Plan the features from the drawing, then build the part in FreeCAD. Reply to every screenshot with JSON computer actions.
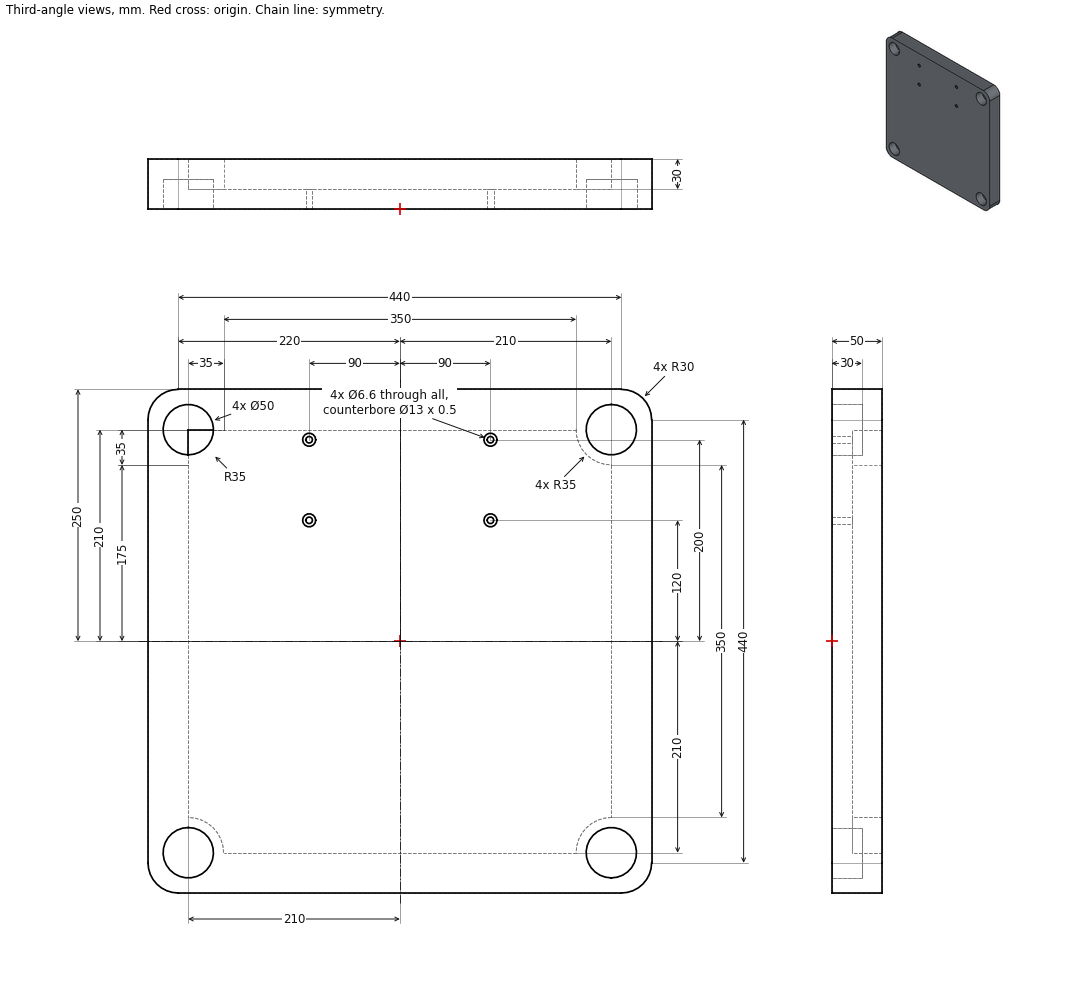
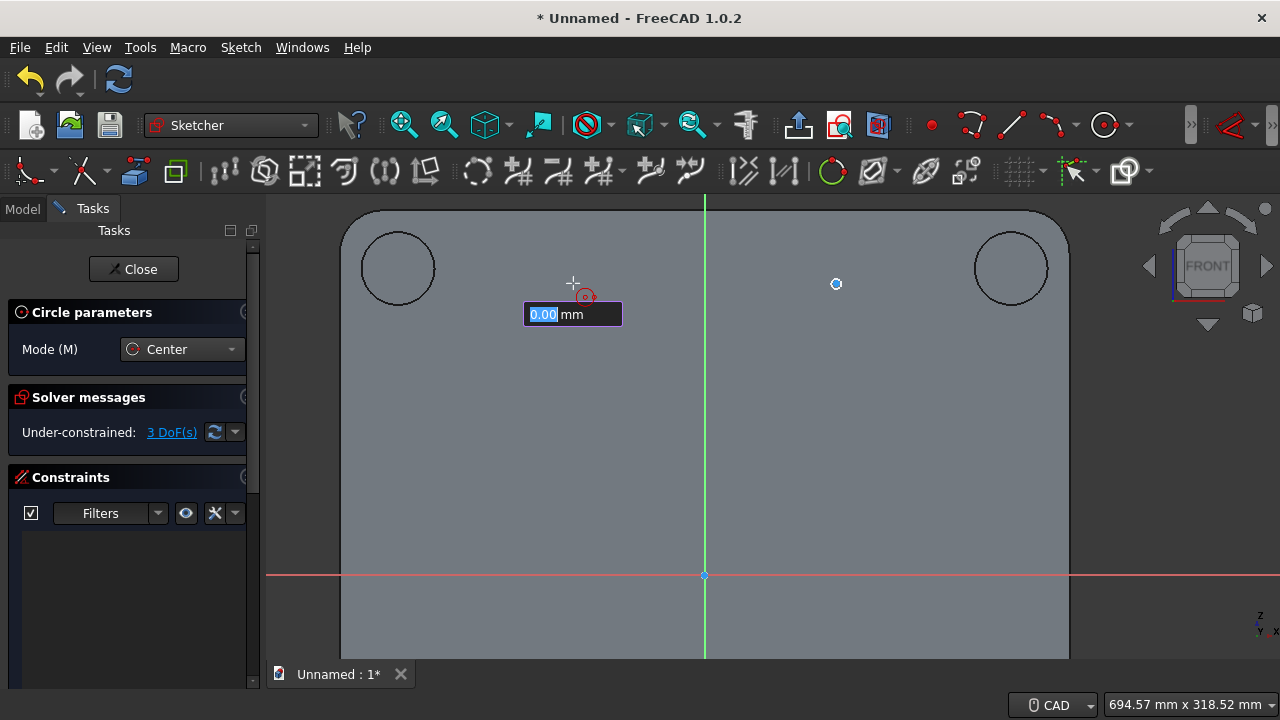
{"action": "scroll", "coordinate": [577, 280], "scroll_direction": "up", "scroll_amount": 6}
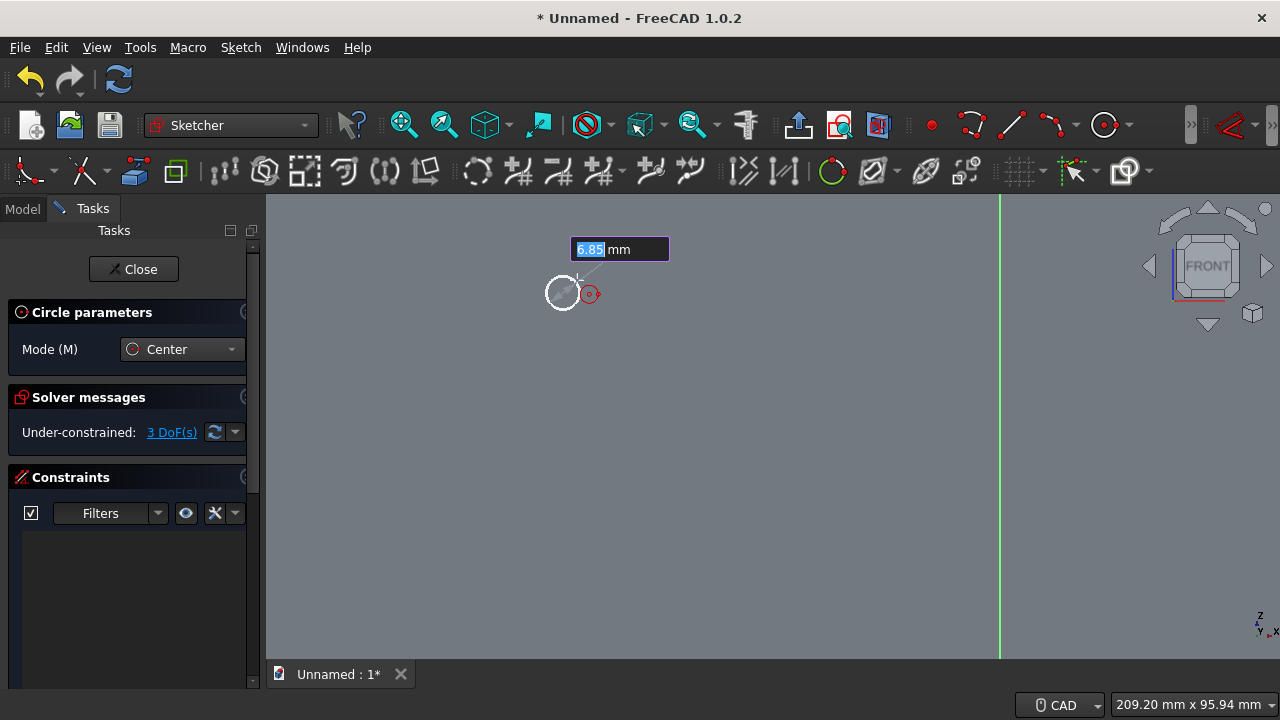
{"action": "left_click", "coordinate": [575, 279]}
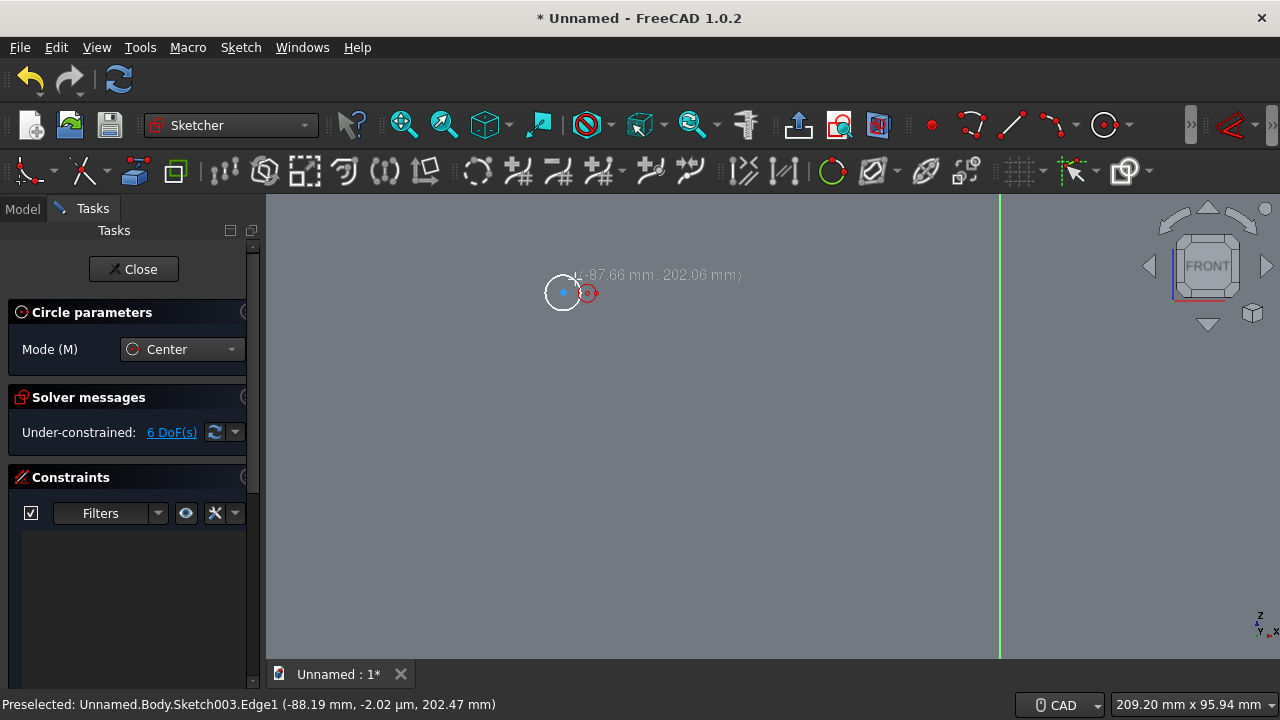
{"action": "scroll", "coordinate": [577, 280], "scroll_direction": "down", "scroll_amount": 6}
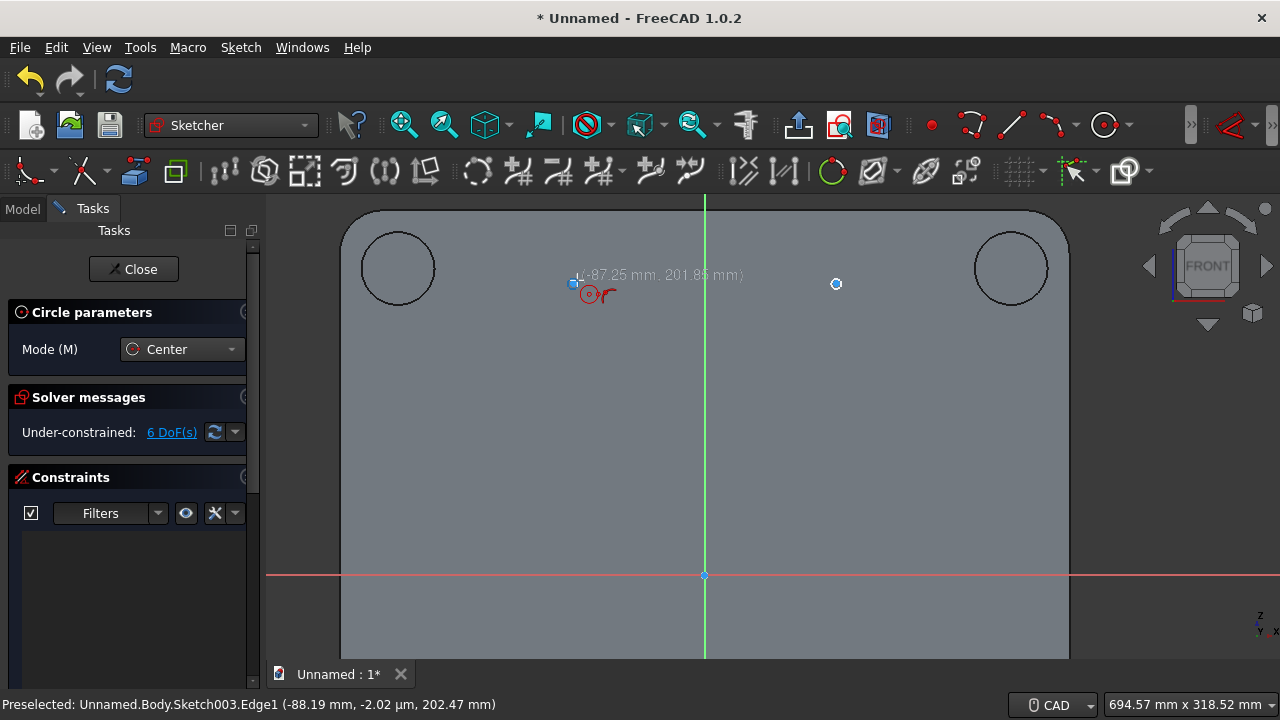
{"action": "scroll", "coordinate": [836, 400], "scroll_direction": "up", "scroll_amount": 8}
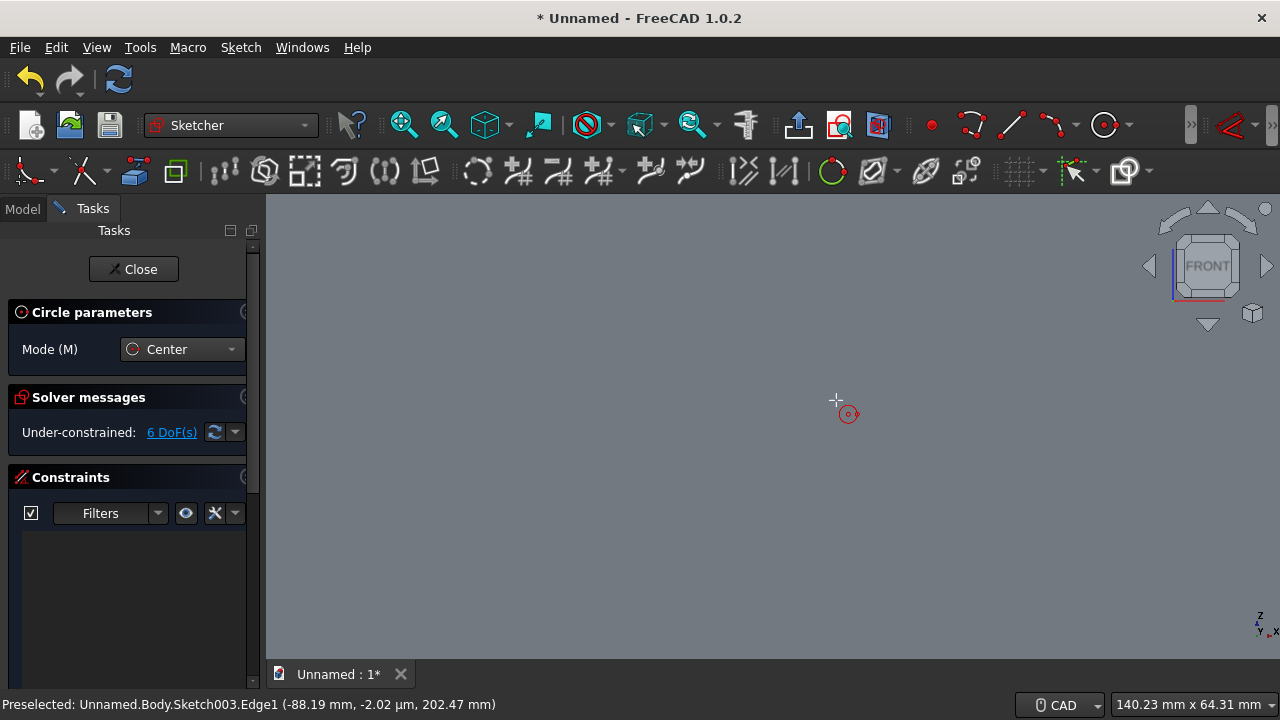
{"action": "scroll", "coordinate": [836, 400], "scroll_direction": "down", "scroll_amount": 8}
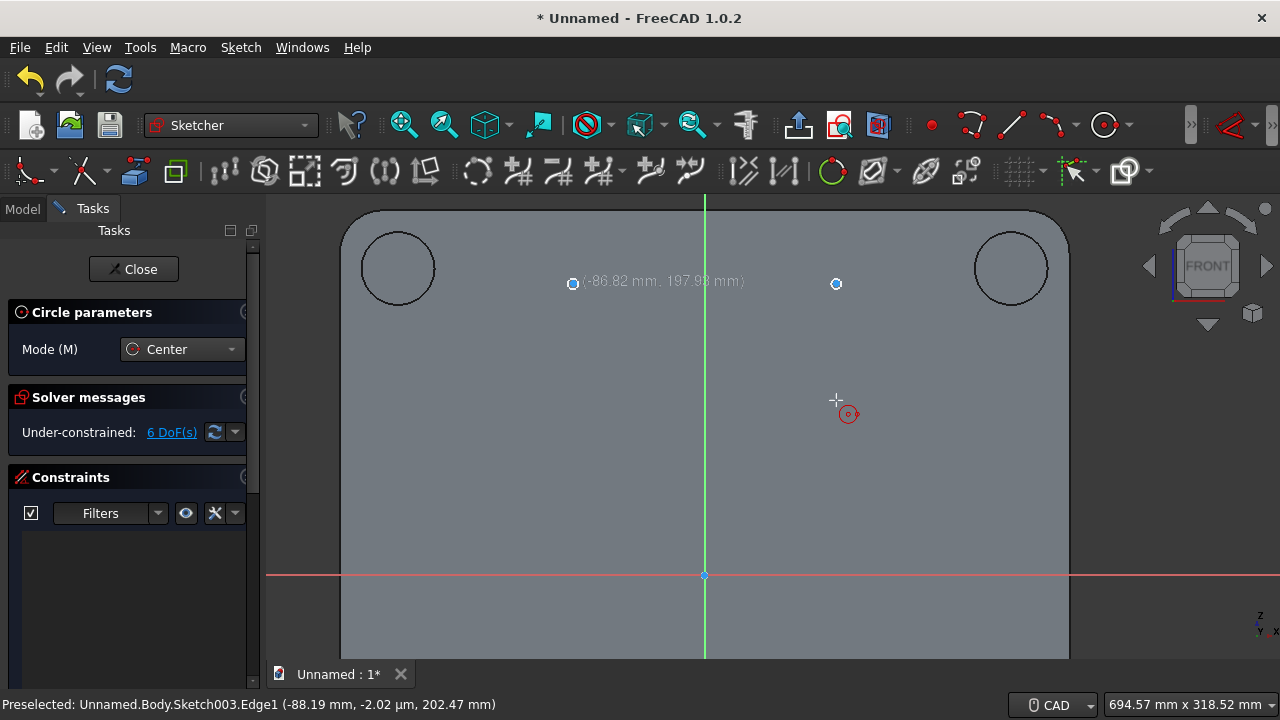
{"action": "left_click", "coordinate": [836, 400]}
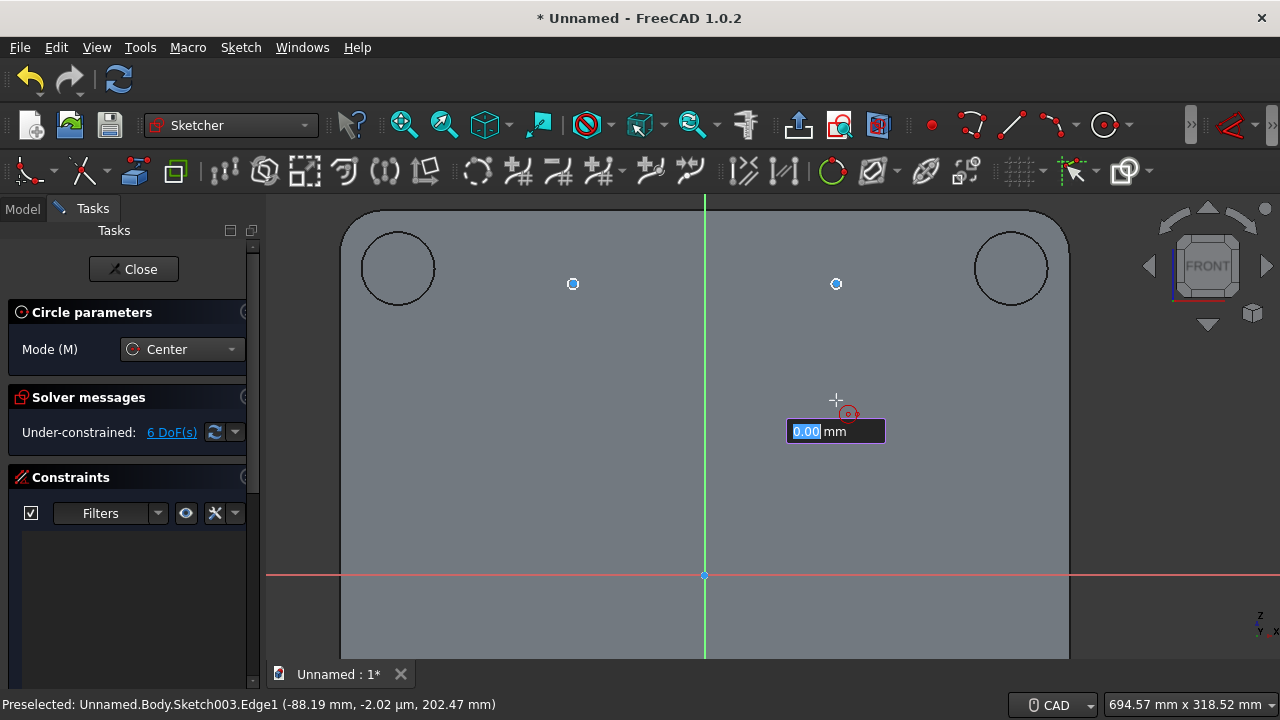
{"action": "scroll", "coordinate": [839, 397], "scroll_direction": "up", "scroll_amount": 6}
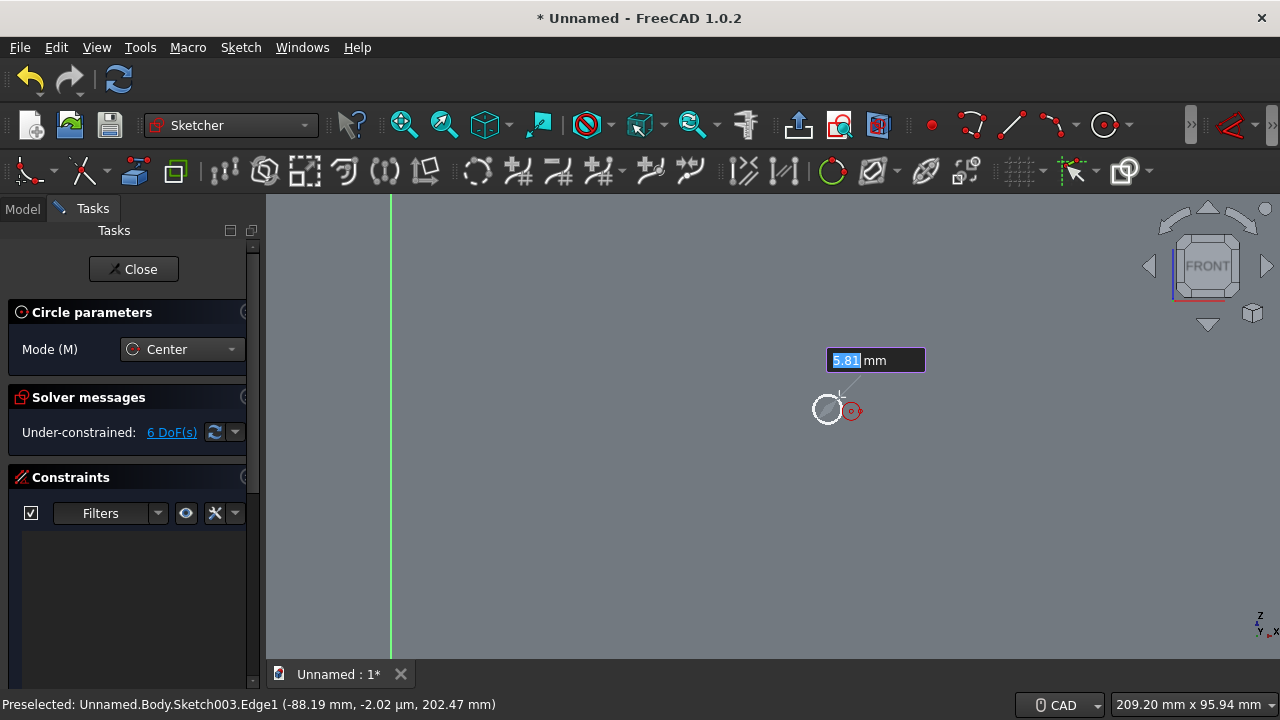
{"action": "left_click", "coordinate": [839, 394]}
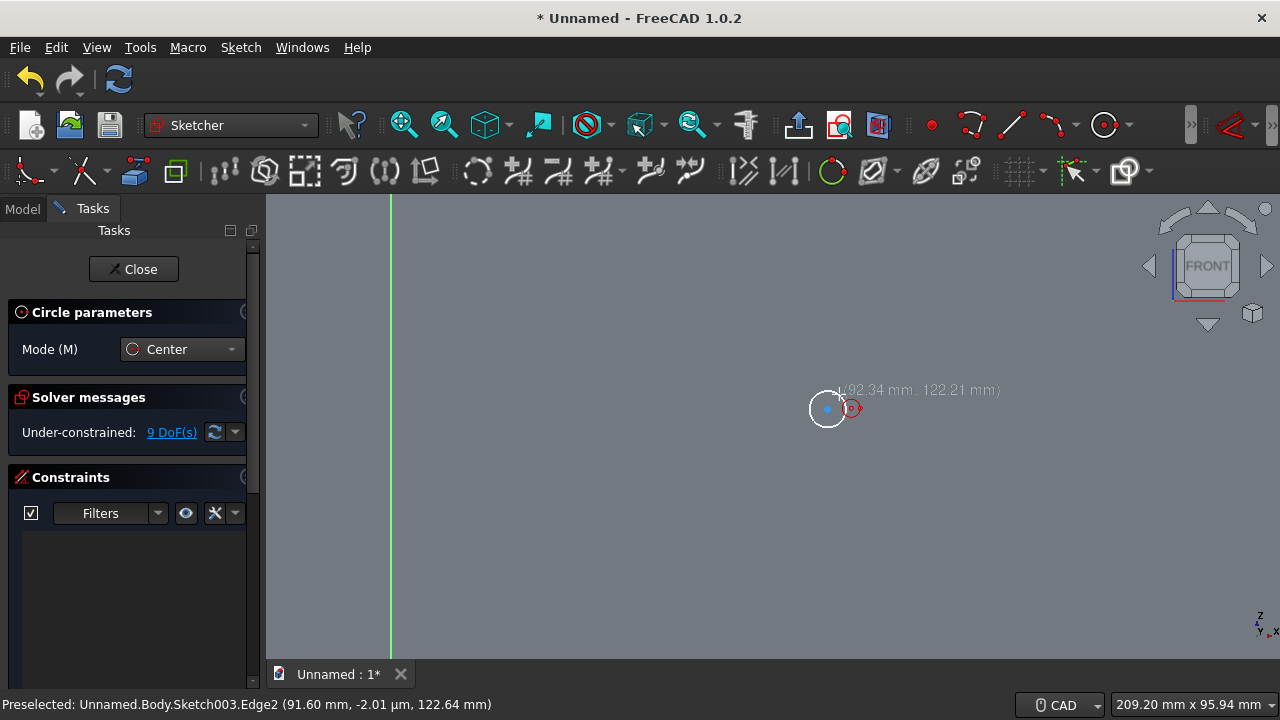
{"action": "scroll", "coordinate": [839, 397], "scroll_direction": "down", "scroll_amount": 6}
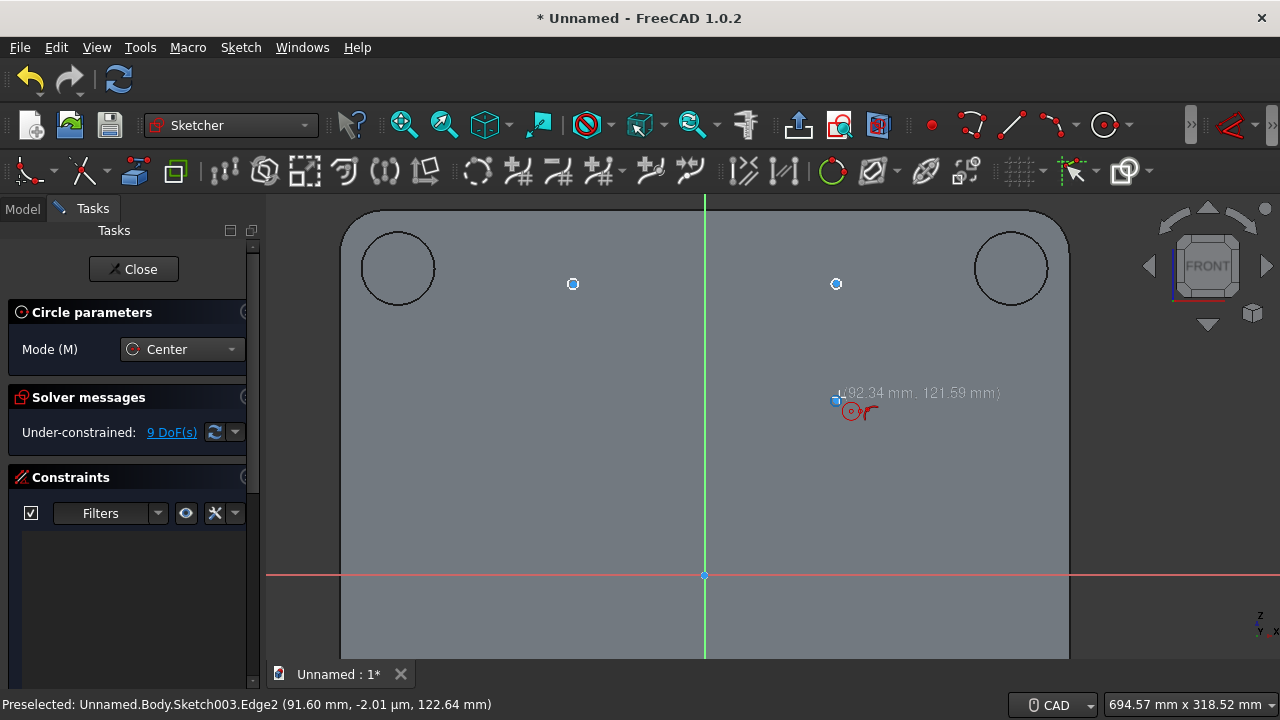
{"action": "scroll", "coordinate": [573, 400], "scroll_direction": "up", "scroll_amount": 8}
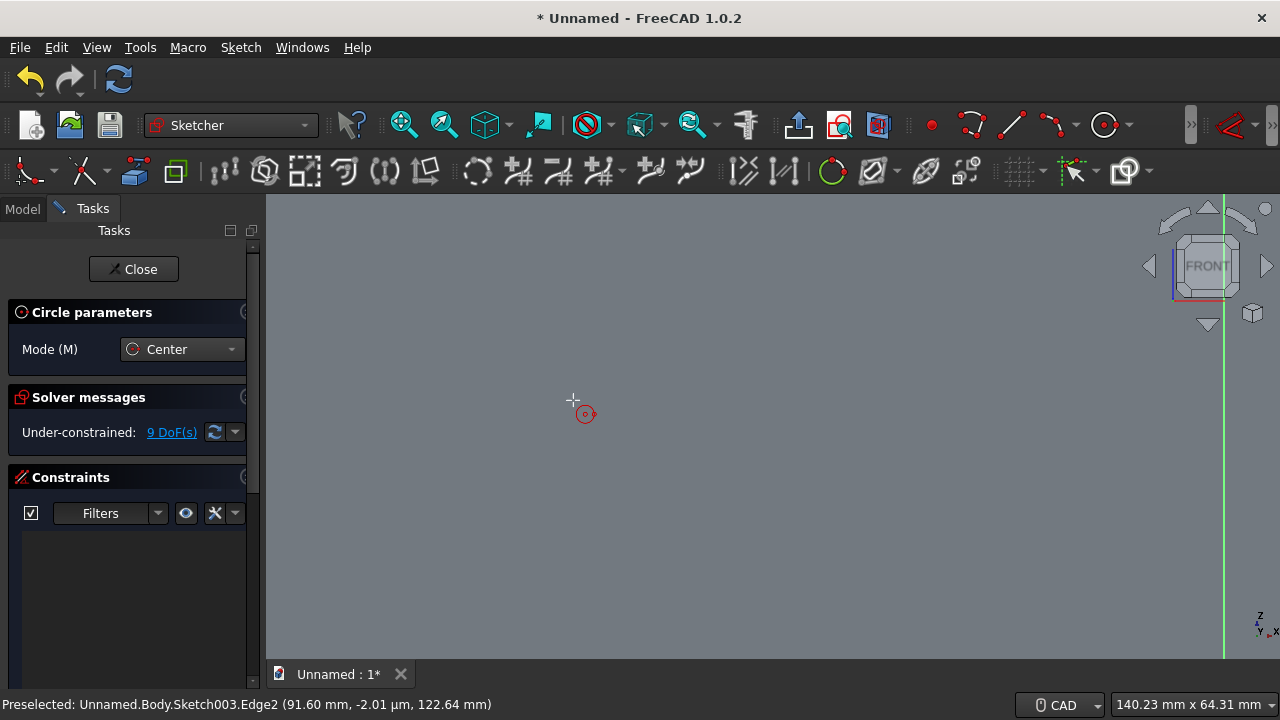
{"action": "scroll", "coordinate": [573, 400], "scroll_direction": "down", "scroll_amount": 8}